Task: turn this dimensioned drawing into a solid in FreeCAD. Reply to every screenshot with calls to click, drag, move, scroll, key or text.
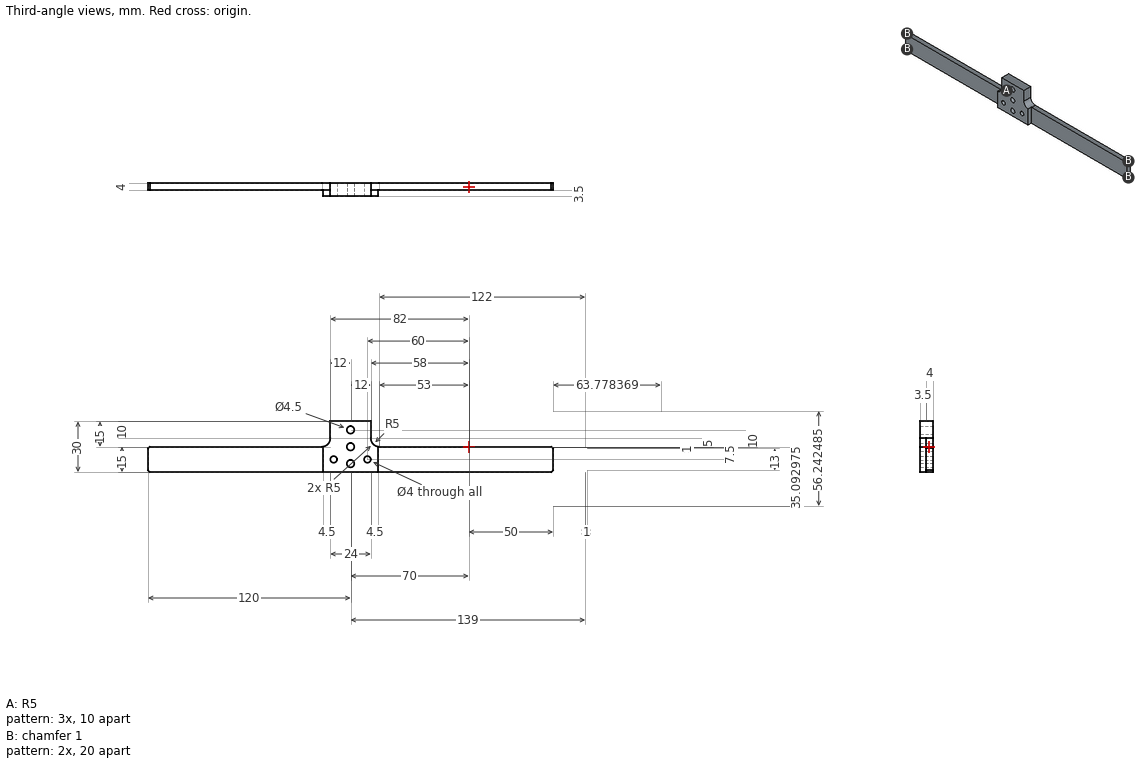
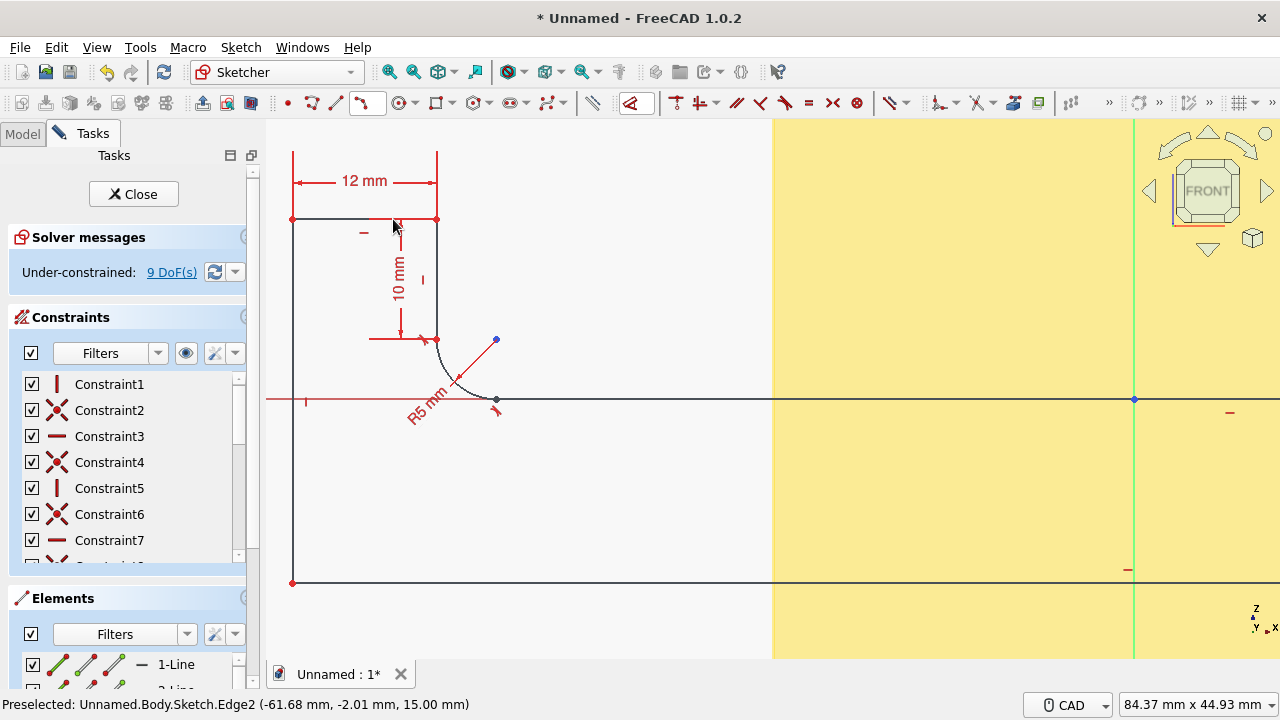
scroll(454, 383, down, 5)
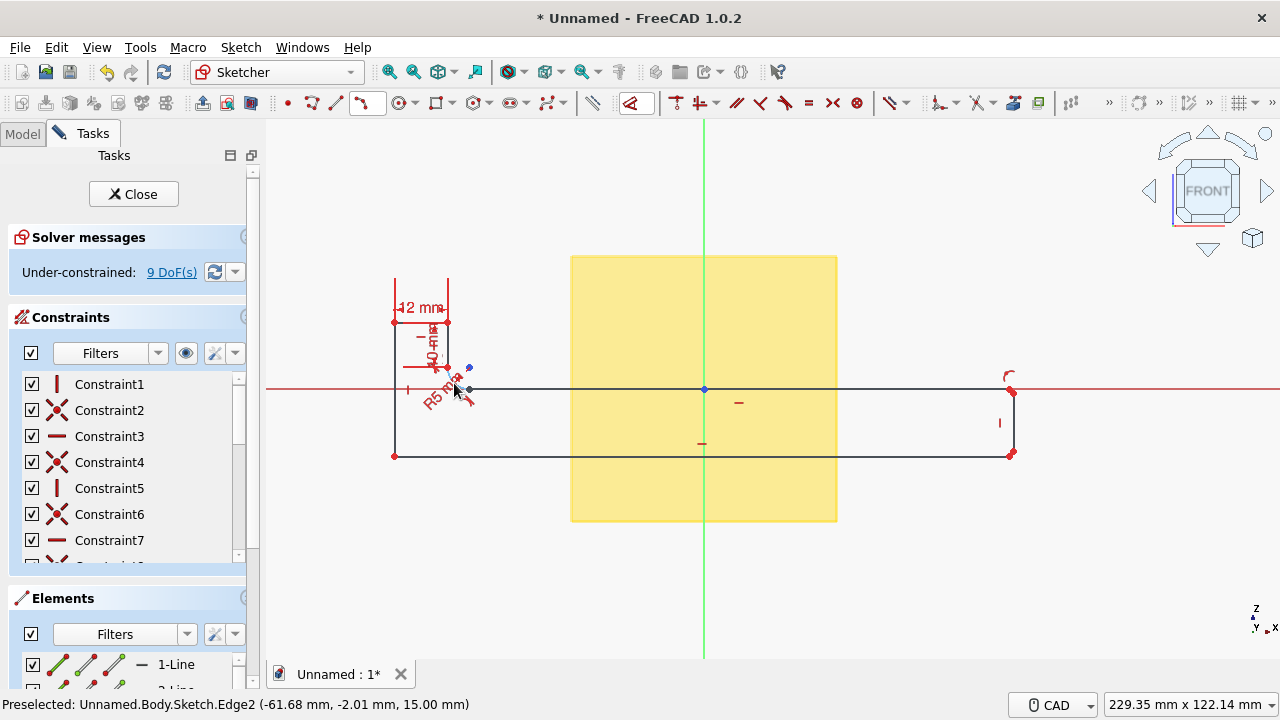
click(395, 363)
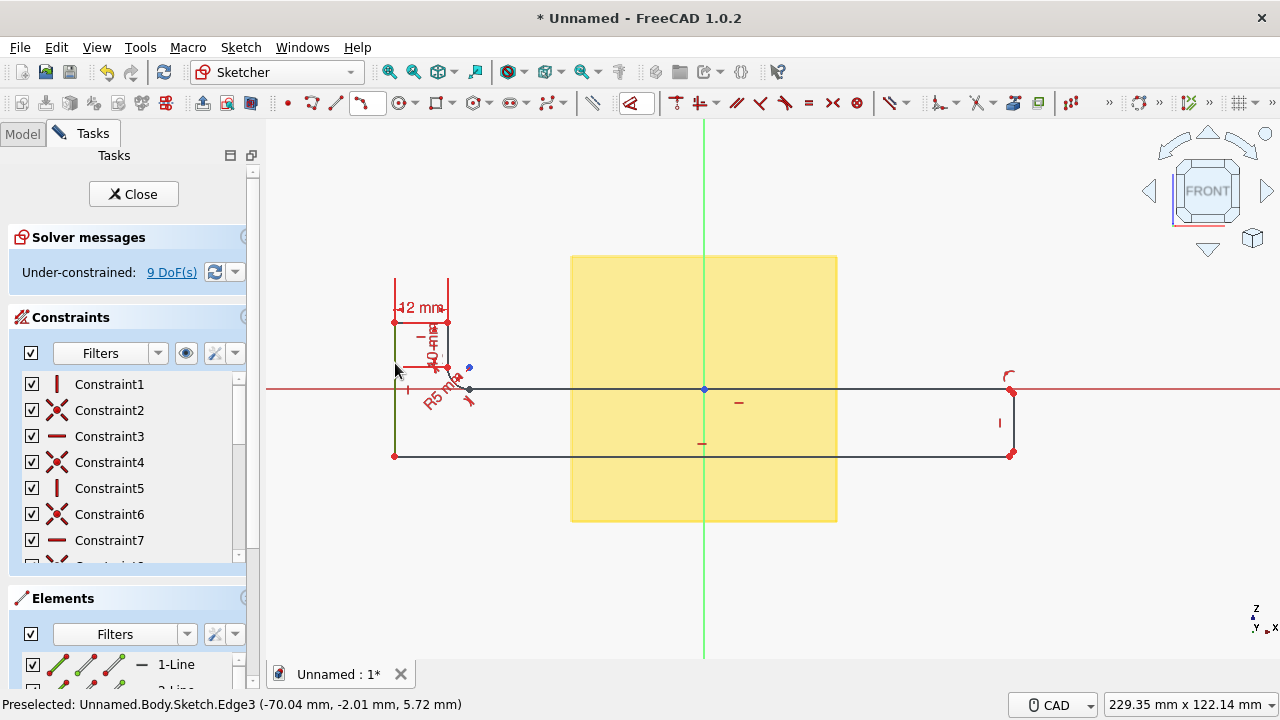
click(648, 104)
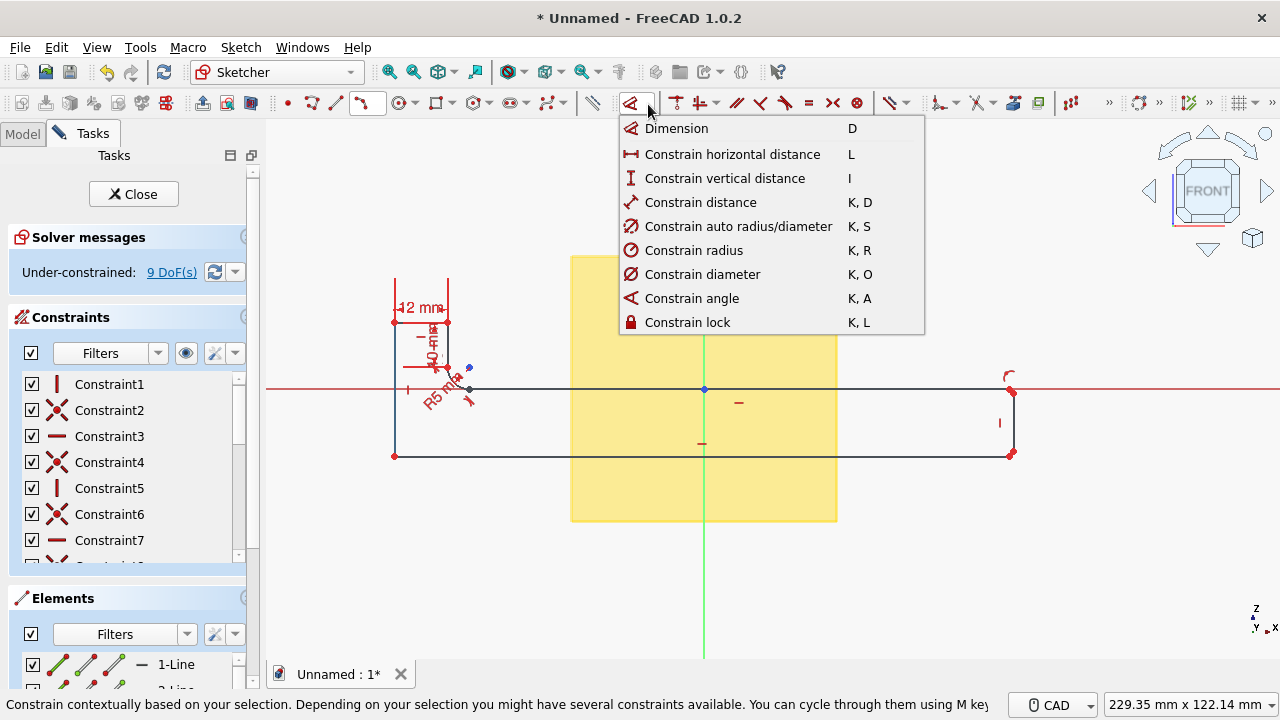
click(772, 178)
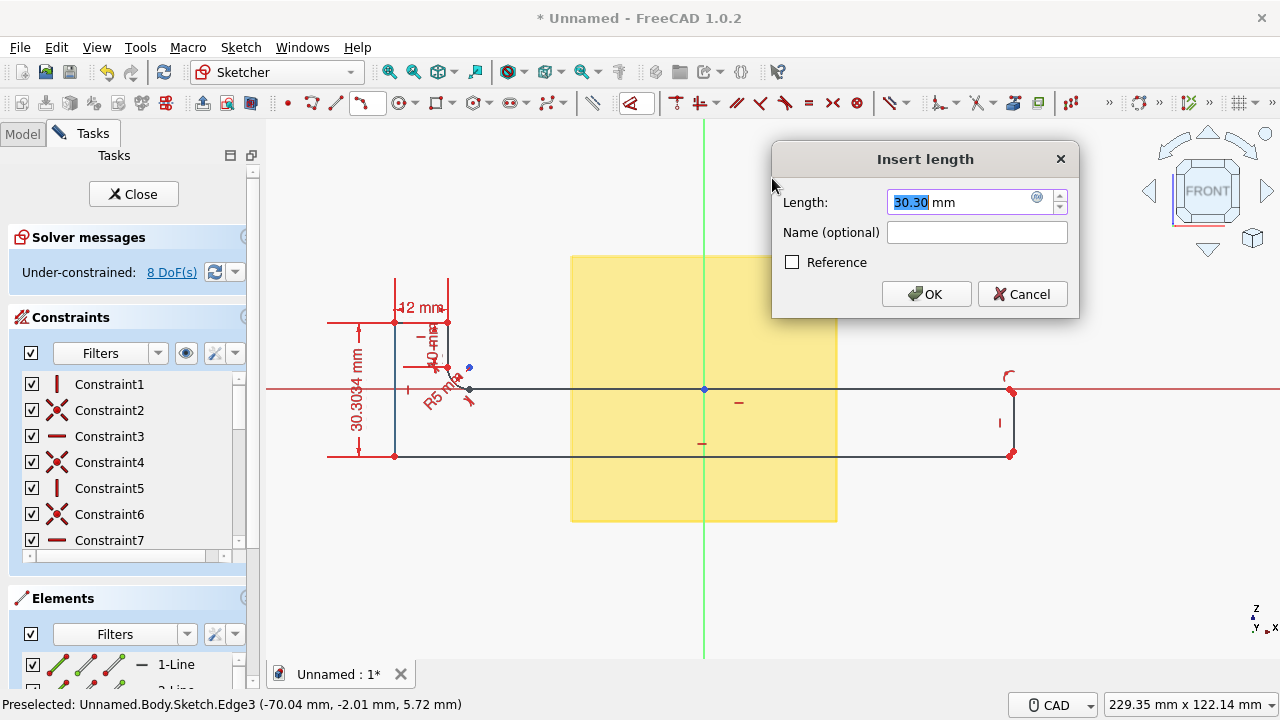
text(30)
key(Return)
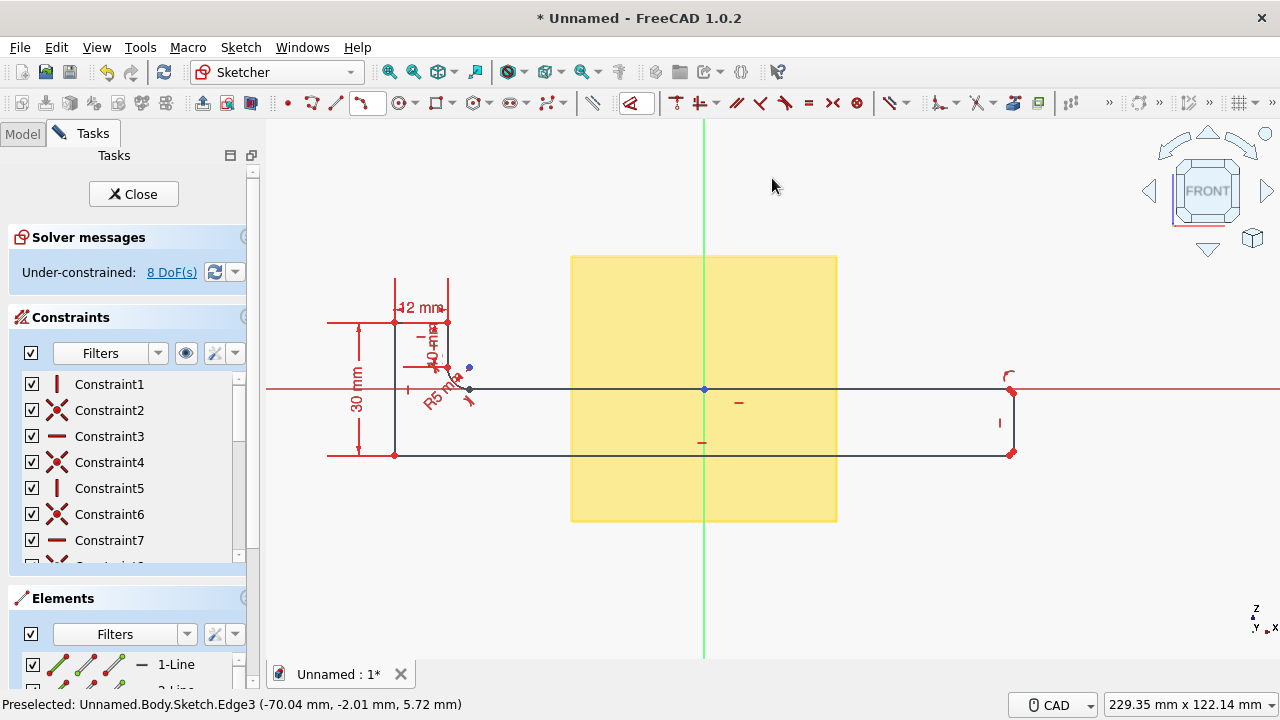
click(1014, 434)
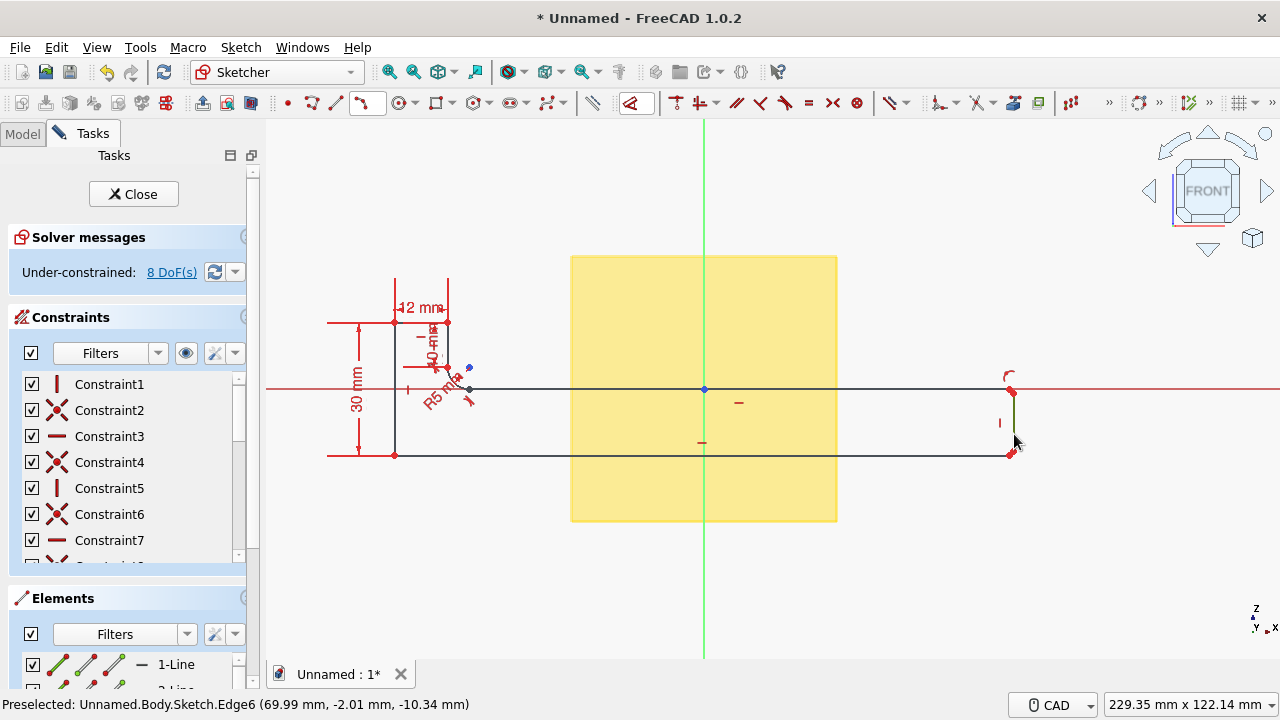
key(i)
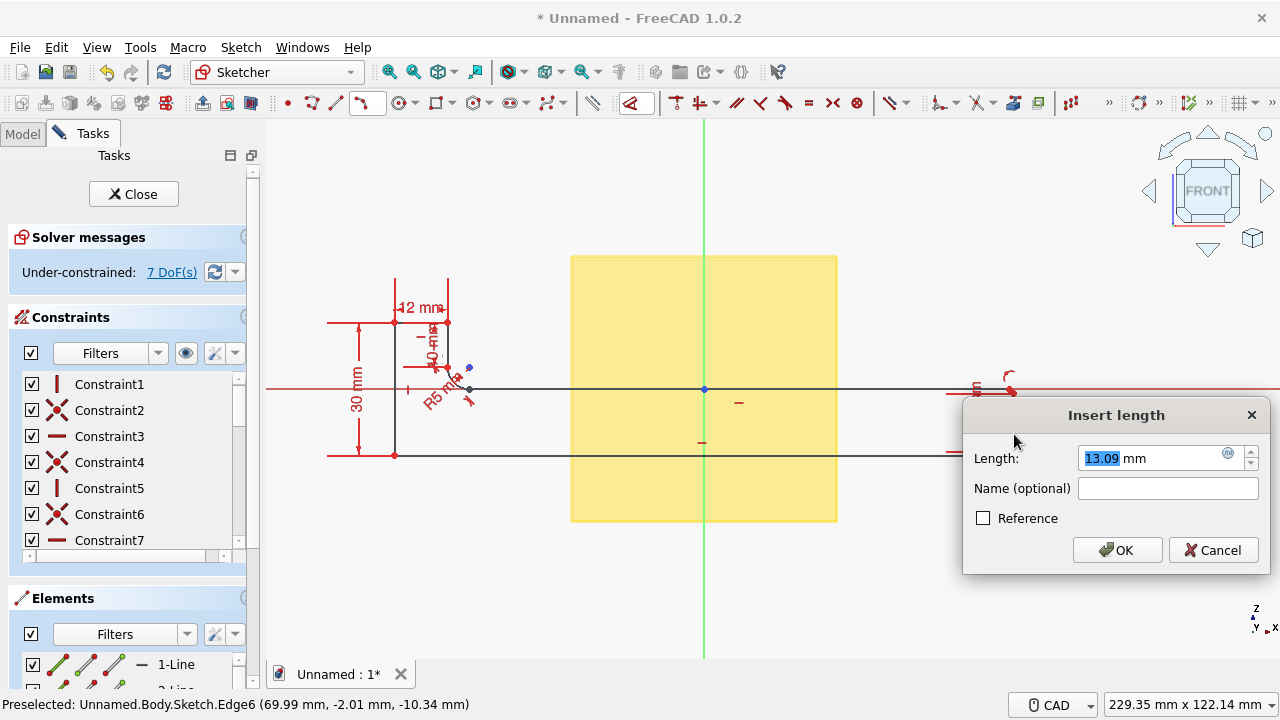
text(13)
key(Return)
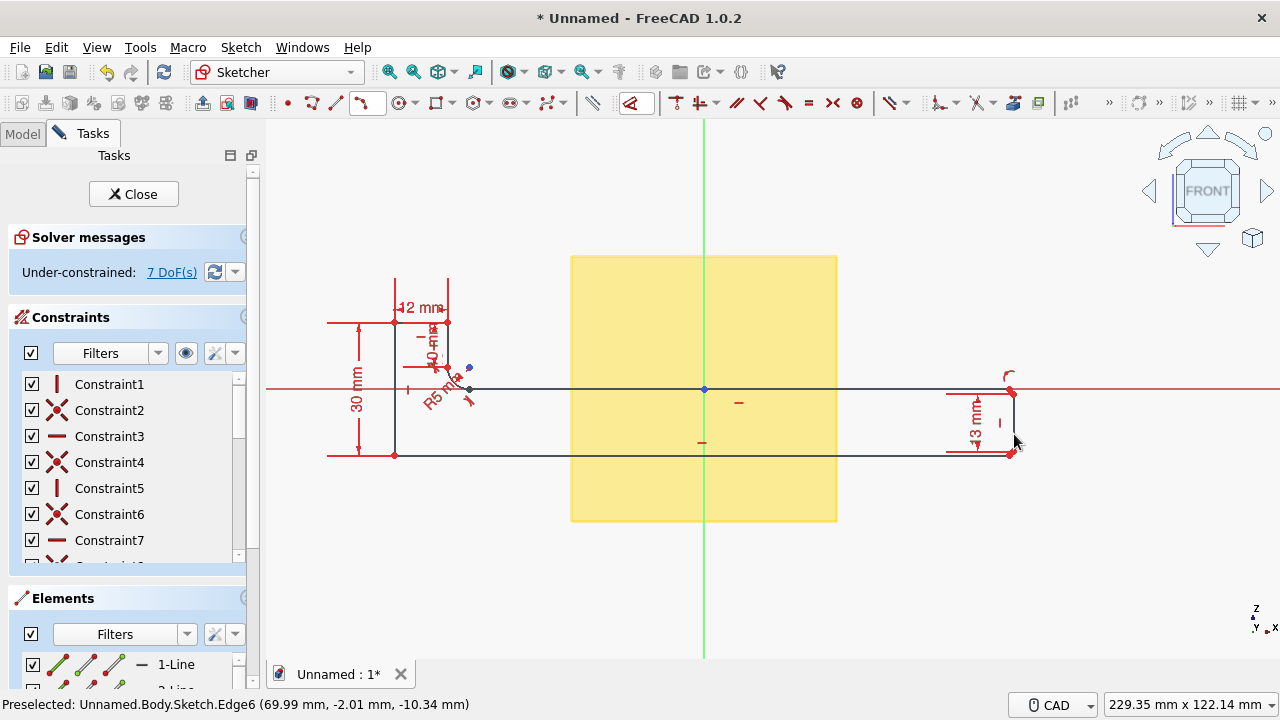
scroll(1014, 394, up, 11)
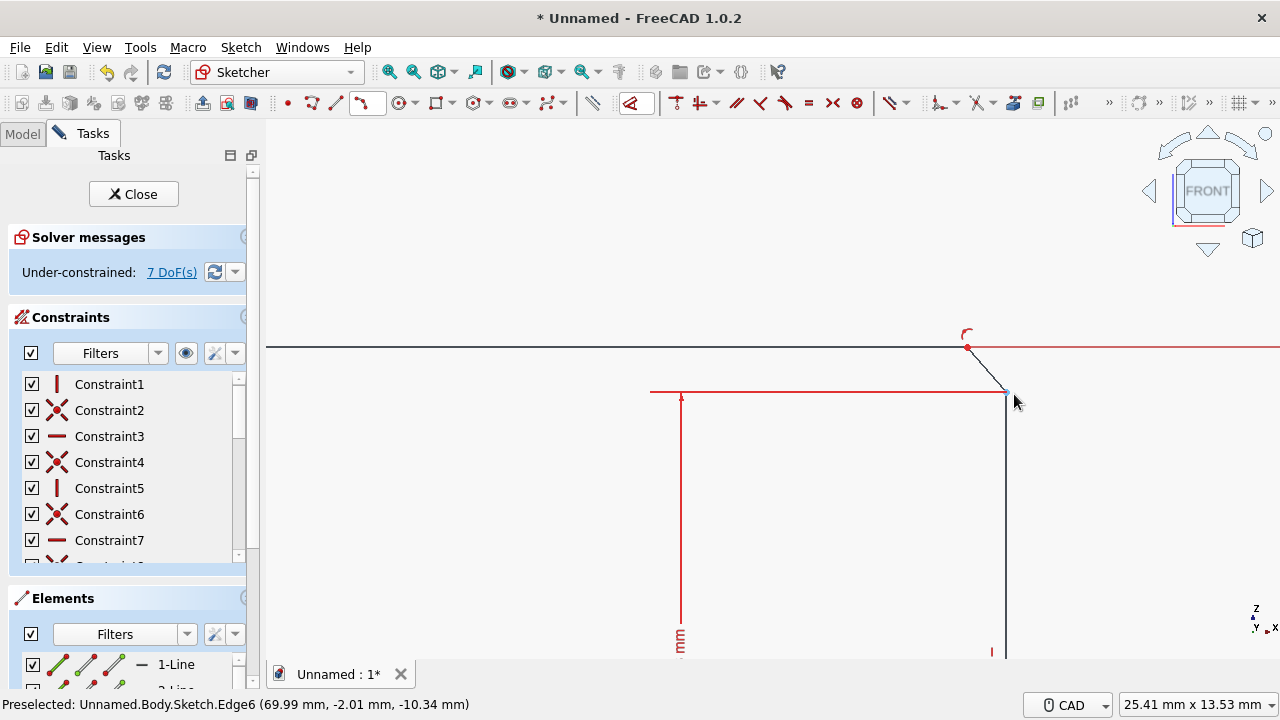
click(1006, 392)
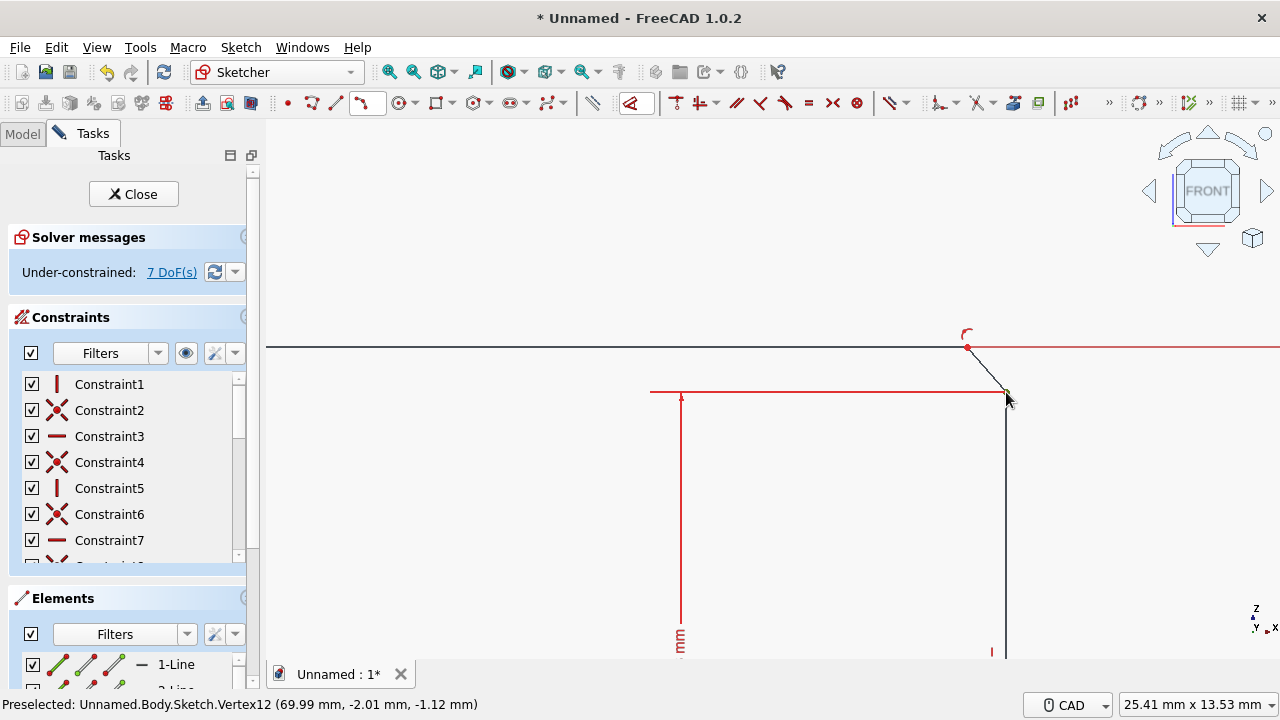
click(648, 104)